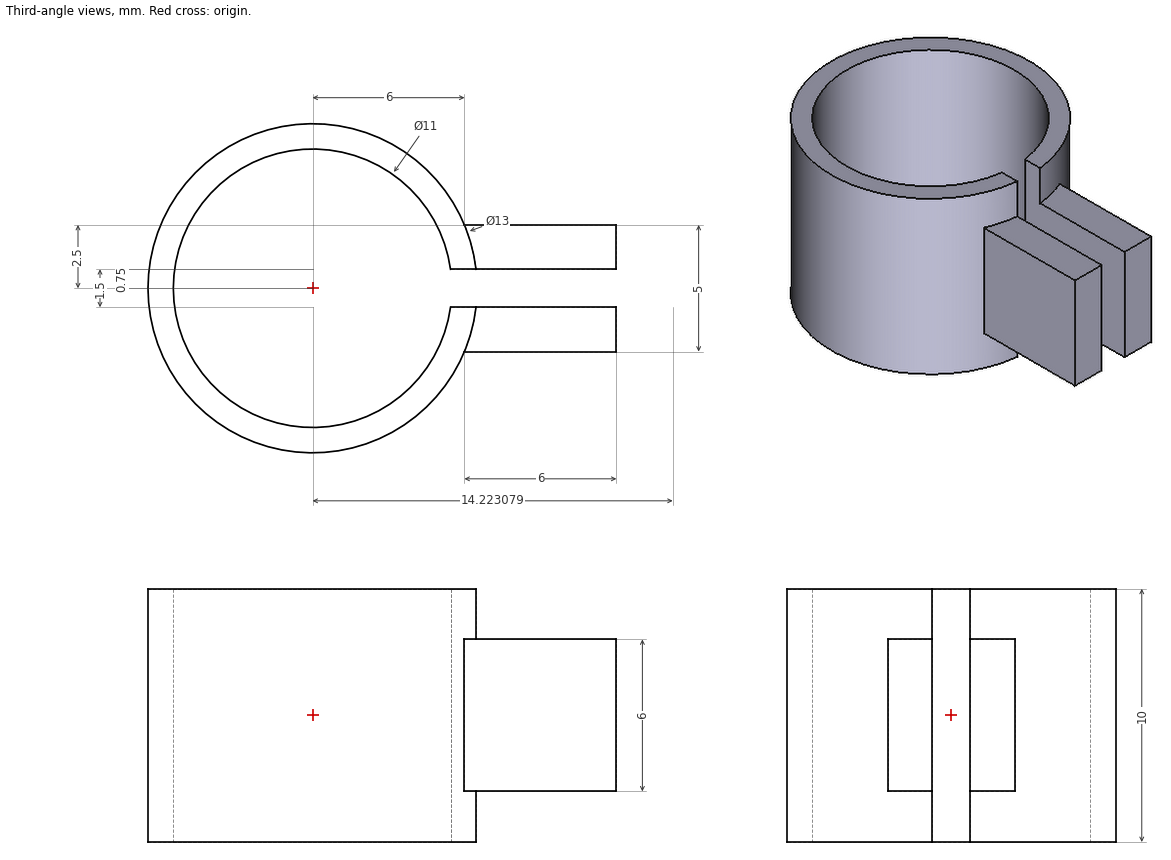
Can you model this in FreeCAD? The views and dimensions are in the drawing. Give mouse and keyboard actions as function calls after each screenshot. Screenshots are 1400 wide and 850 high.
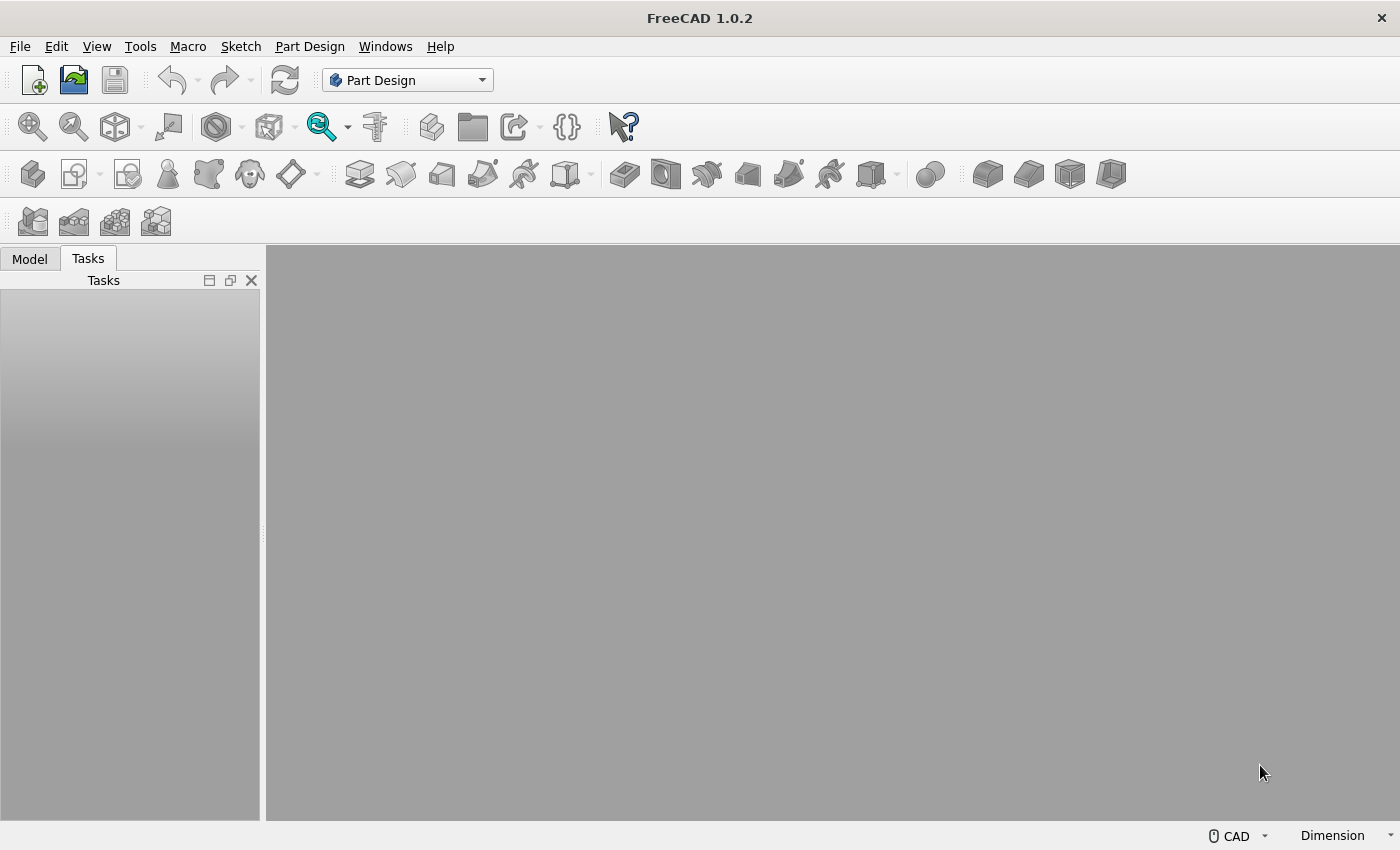
key(ctrl+n)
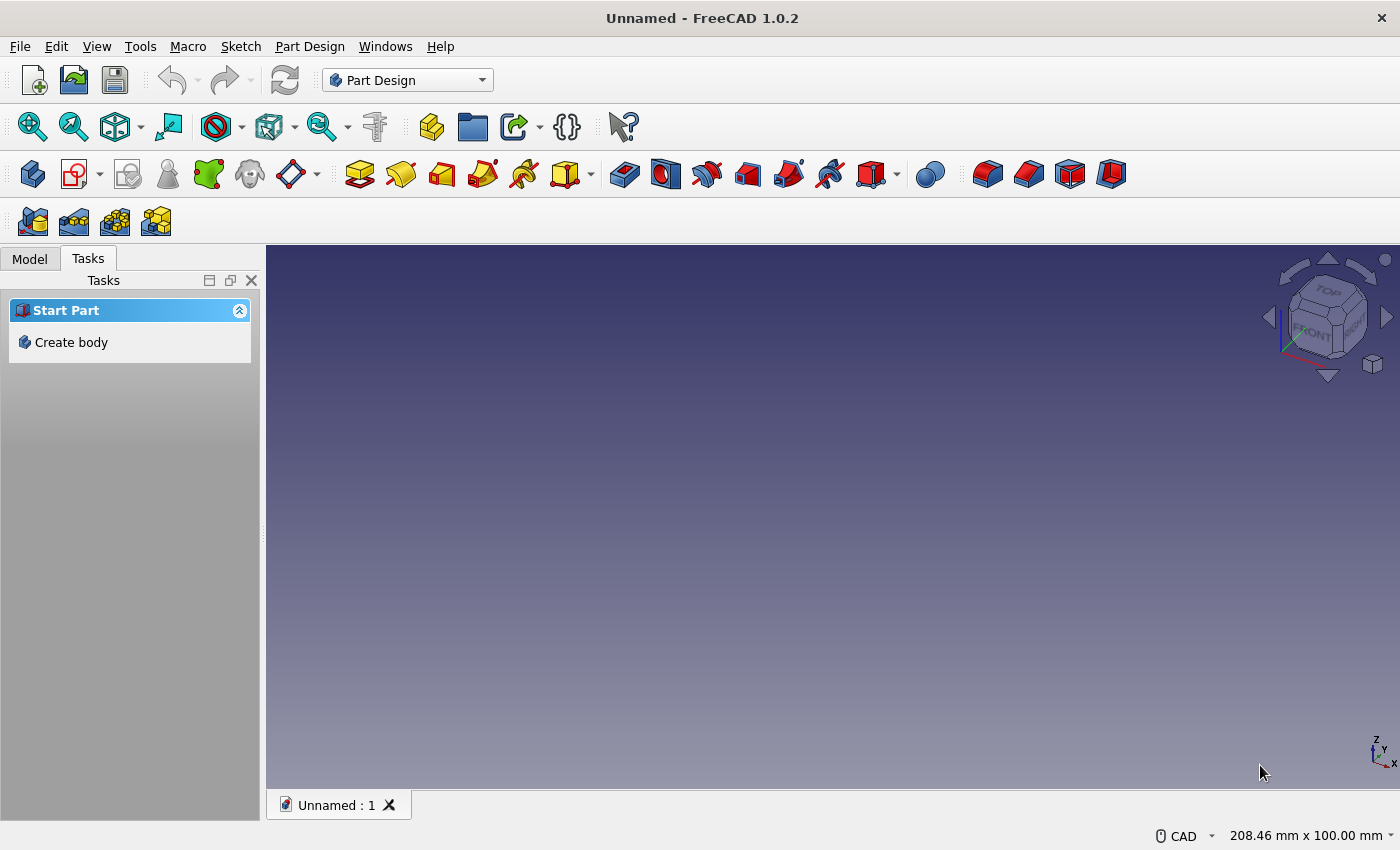
click(74, 174)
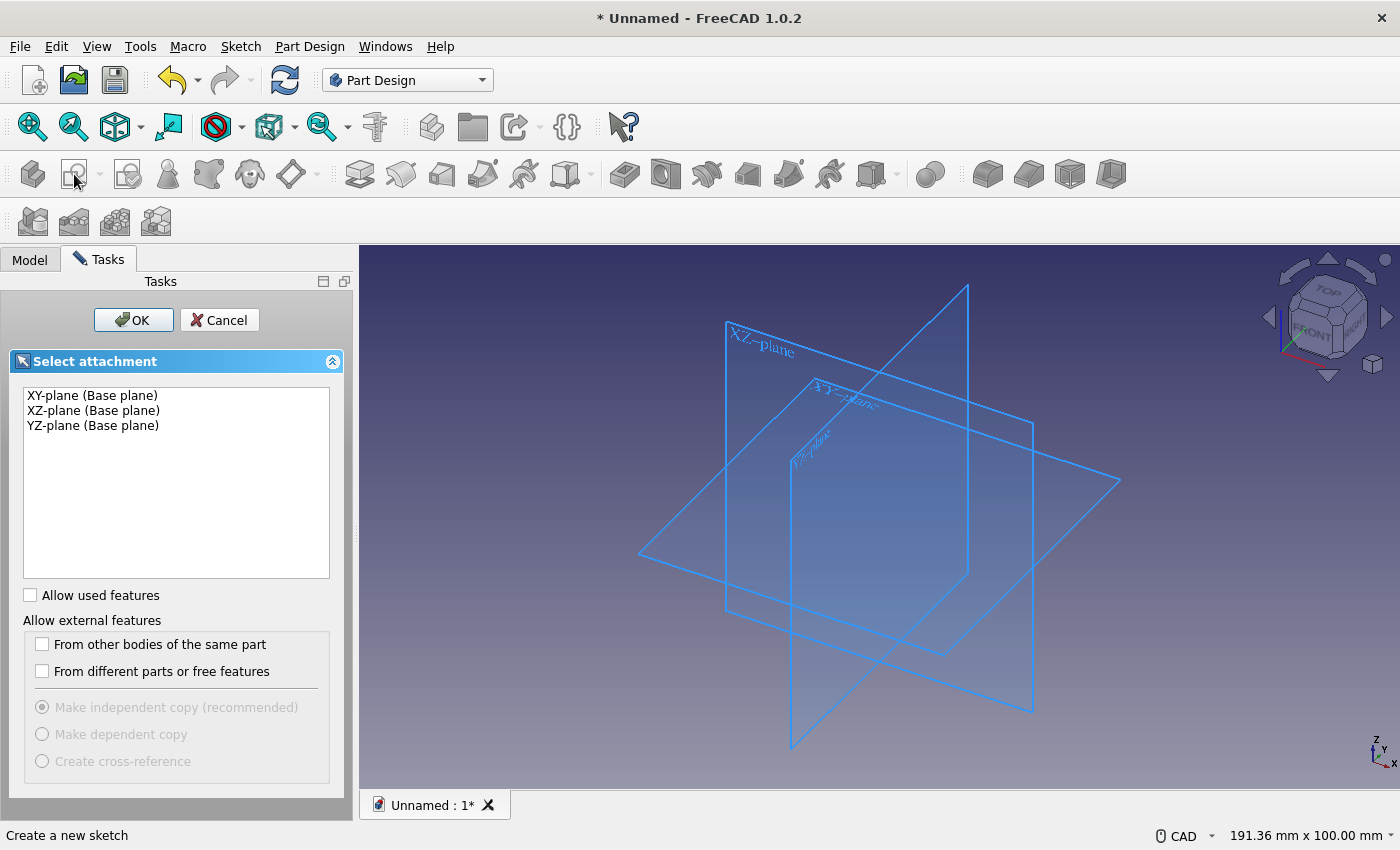
click(84, 396)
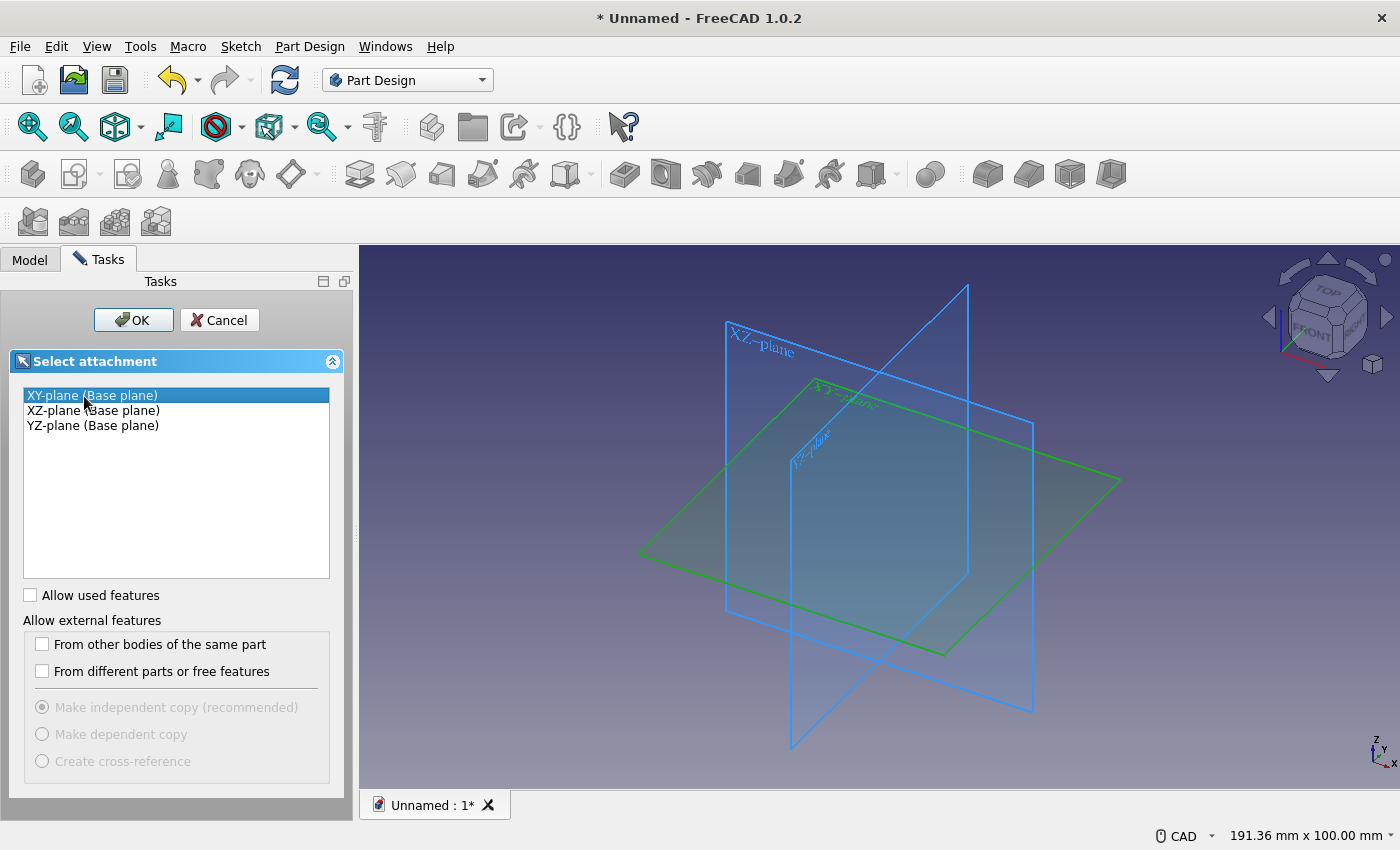
click(134, 320)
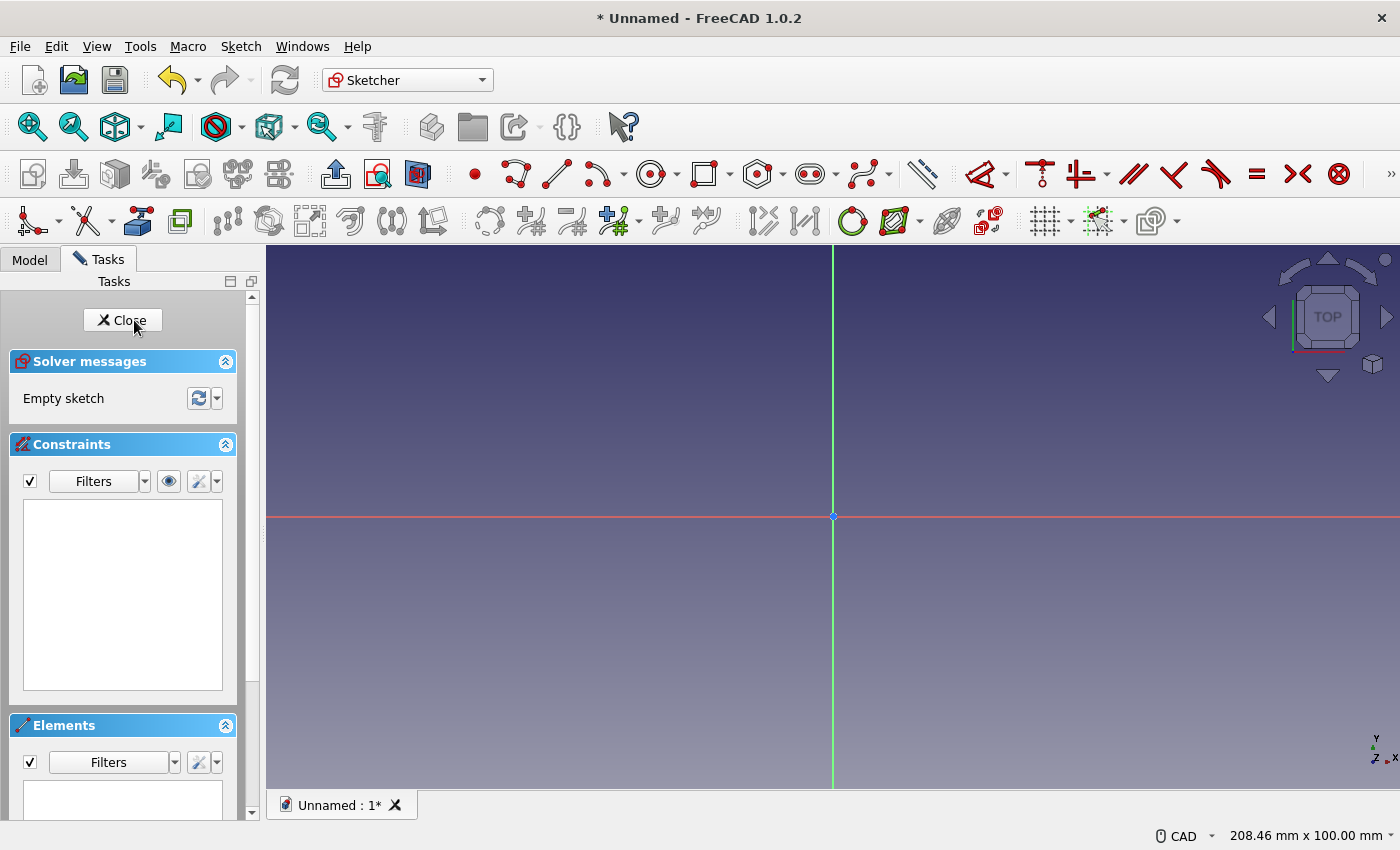
scroll(850, 517, up, 8)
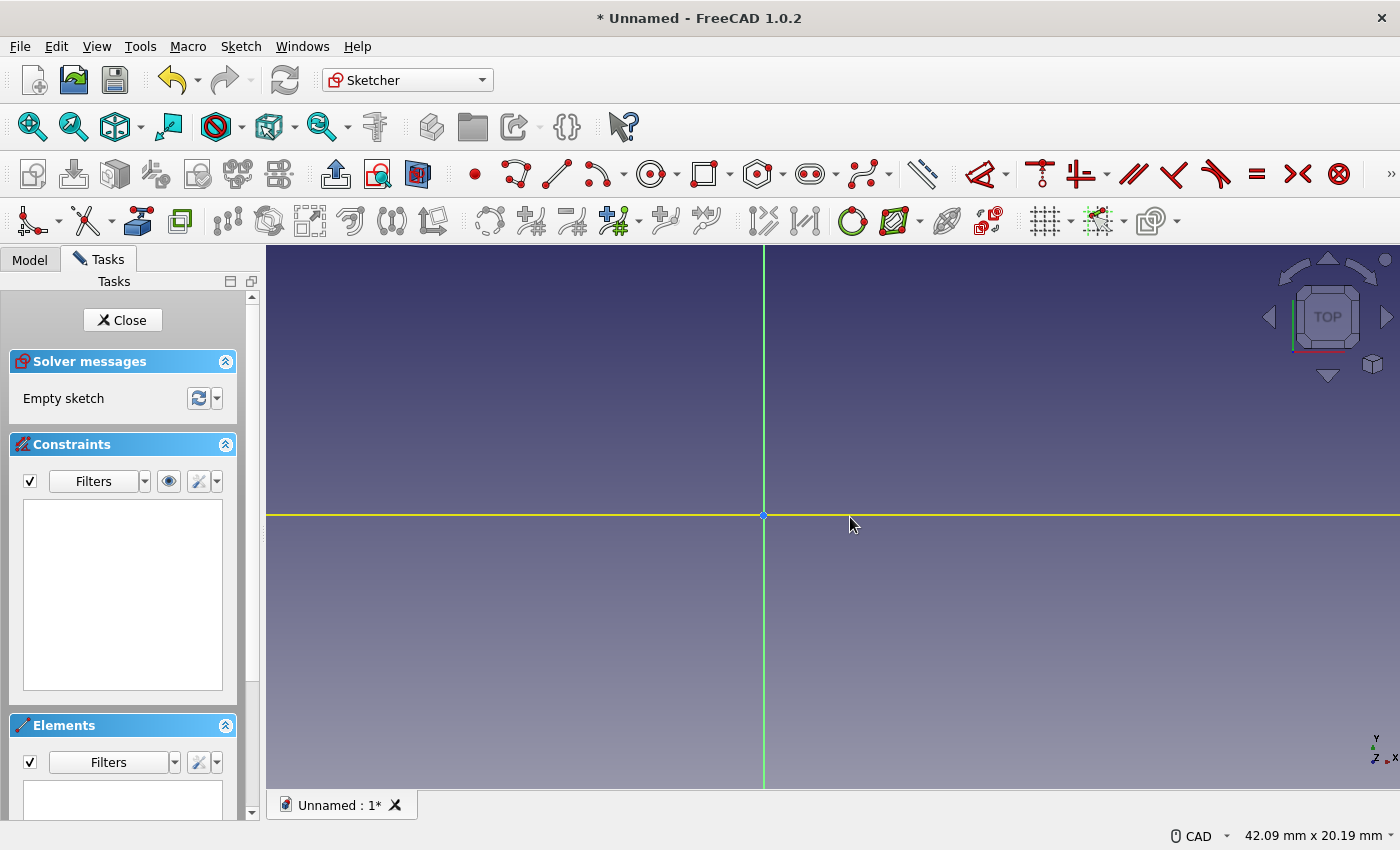
key(g)
key(c)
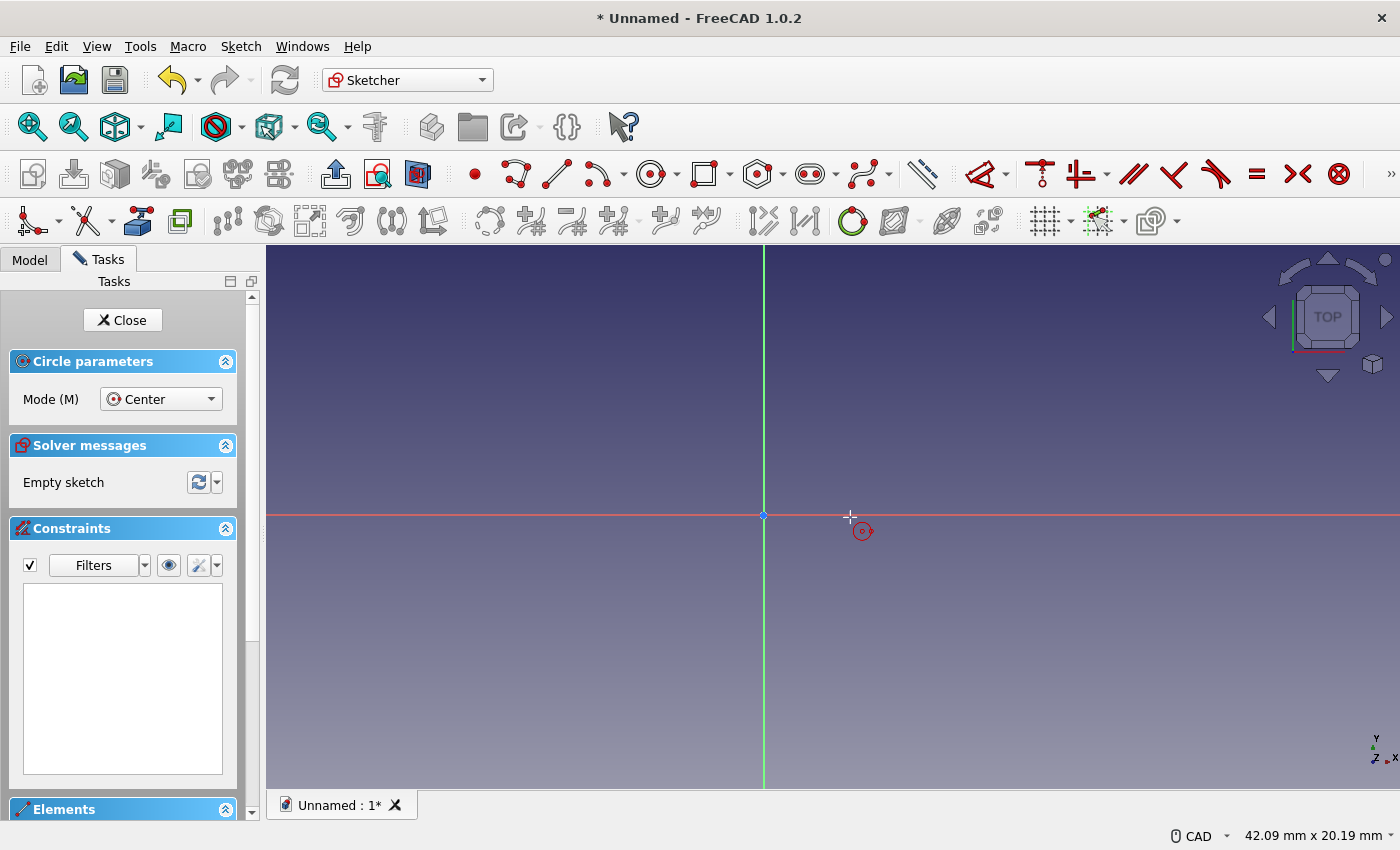
click(764, 515)
click(888, 391)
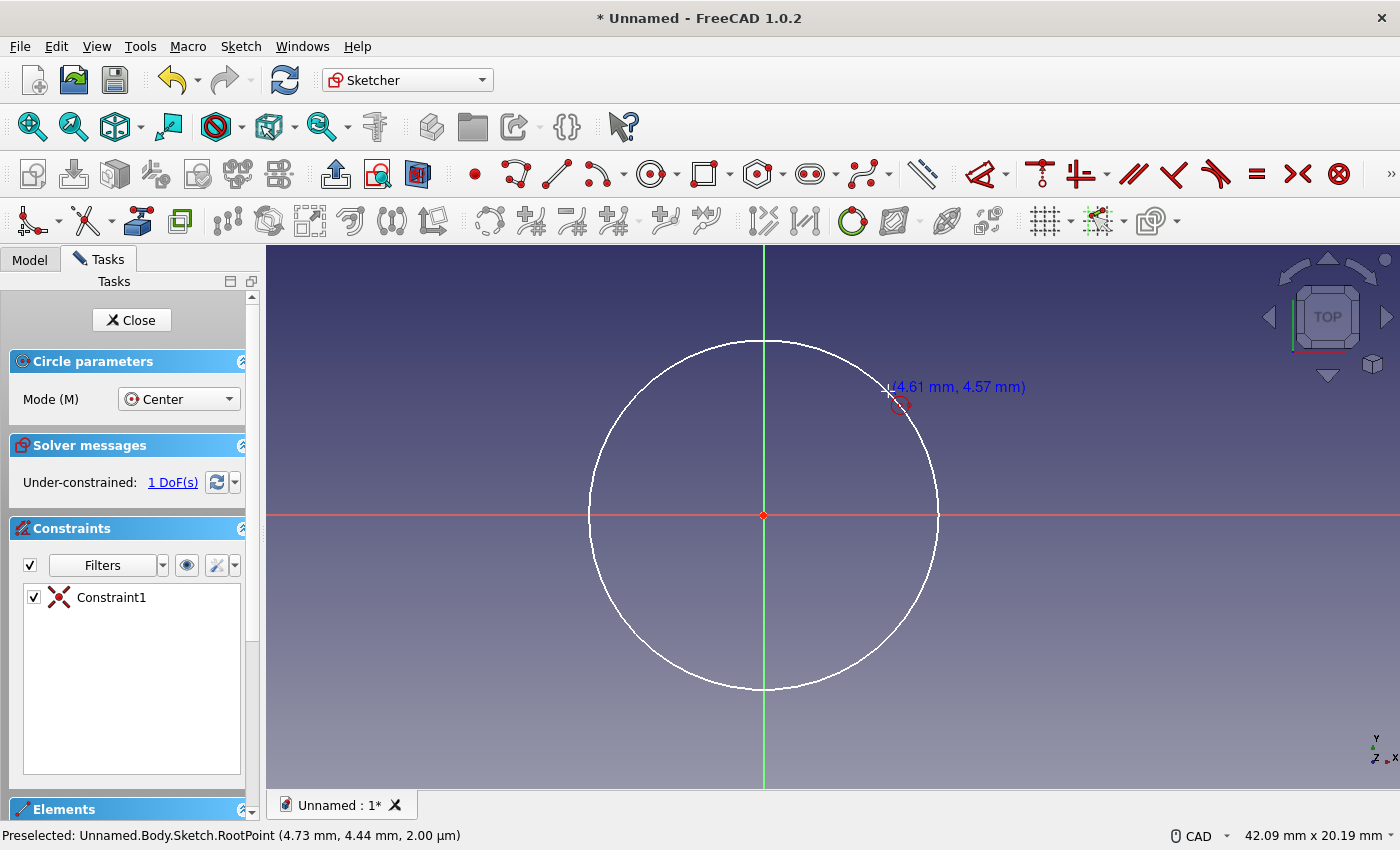
click(764, 515)
click(869, 410)
key(Escape)